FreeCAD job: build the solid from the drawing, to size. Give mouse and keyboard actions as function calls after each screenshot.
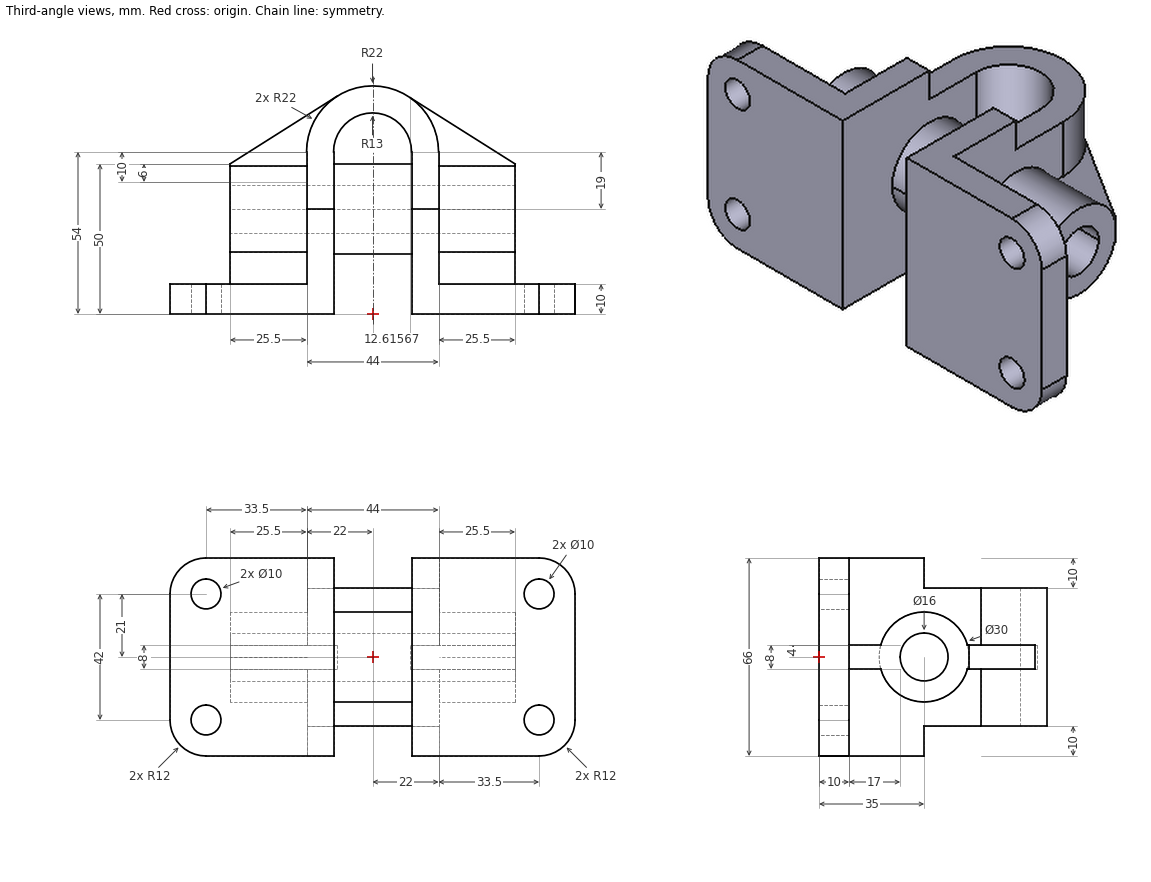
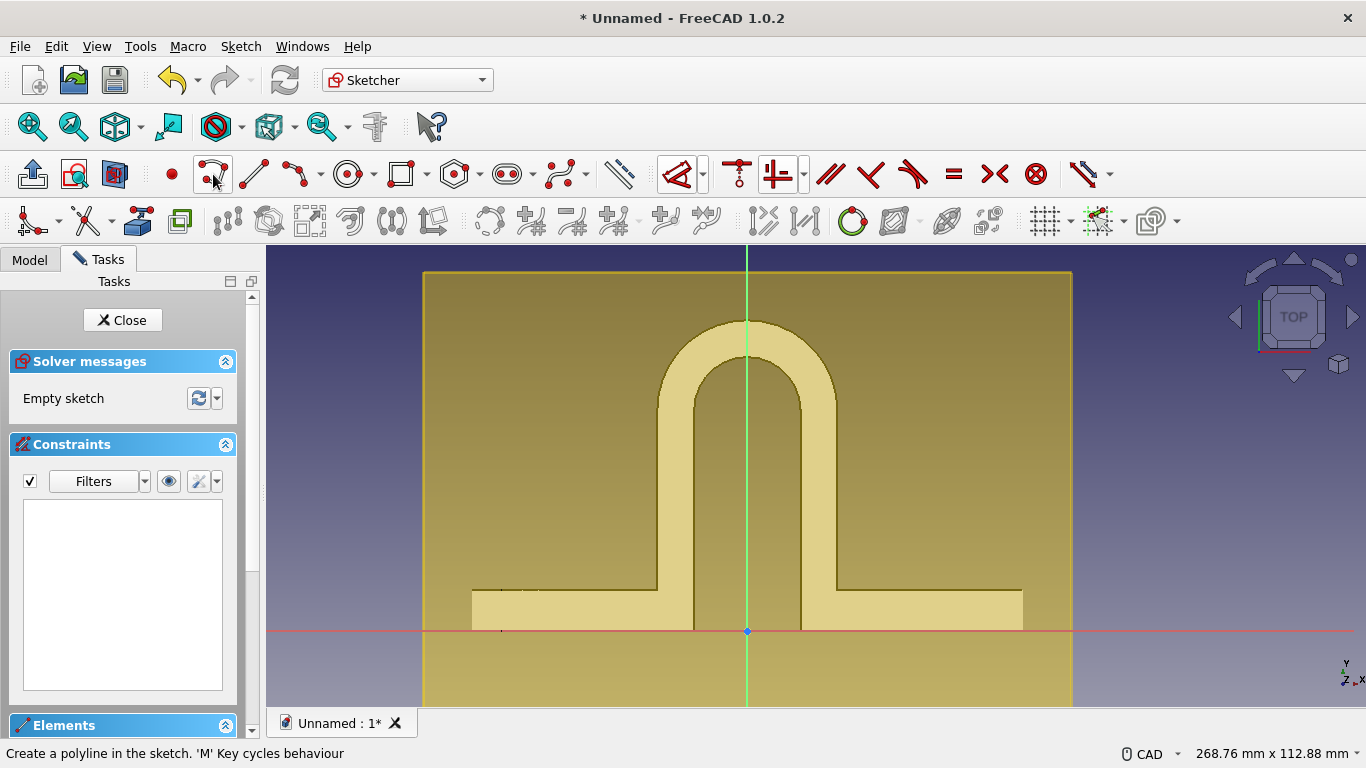
click(694, 410)
click(694, 488)
click(657, 488)
click(657, 410)
right_click(657, 410)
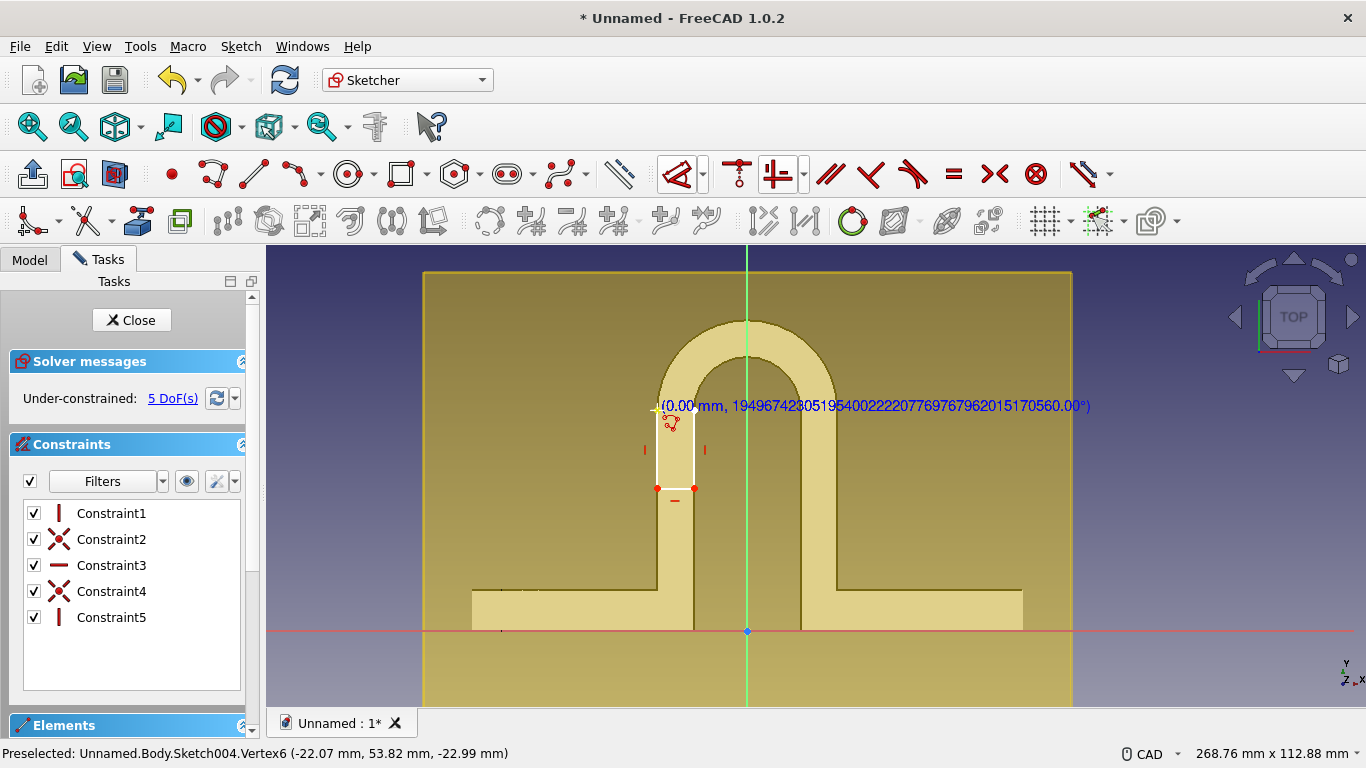
click(837, 410)
click(837, 488)
click(801, 488)
click(801, 410)
right_click(801, 410)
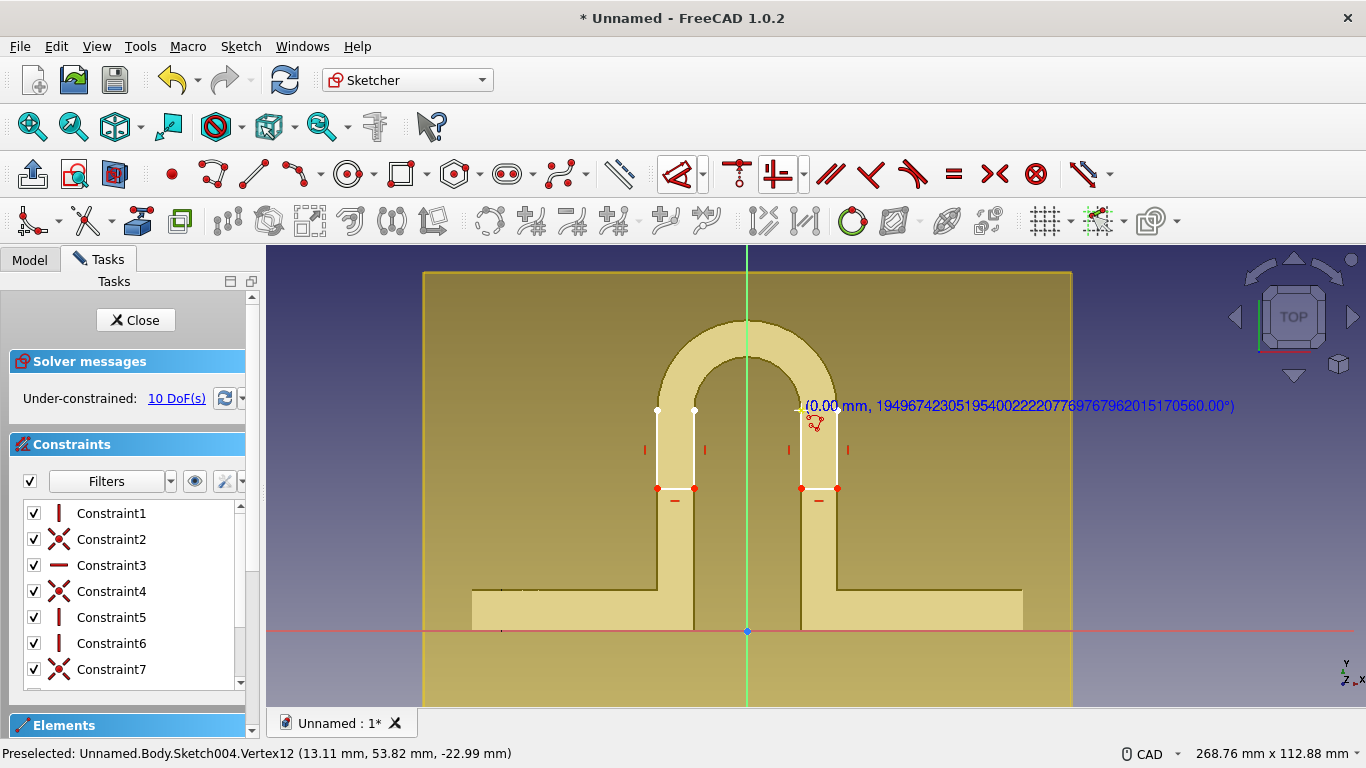
click(294, 174)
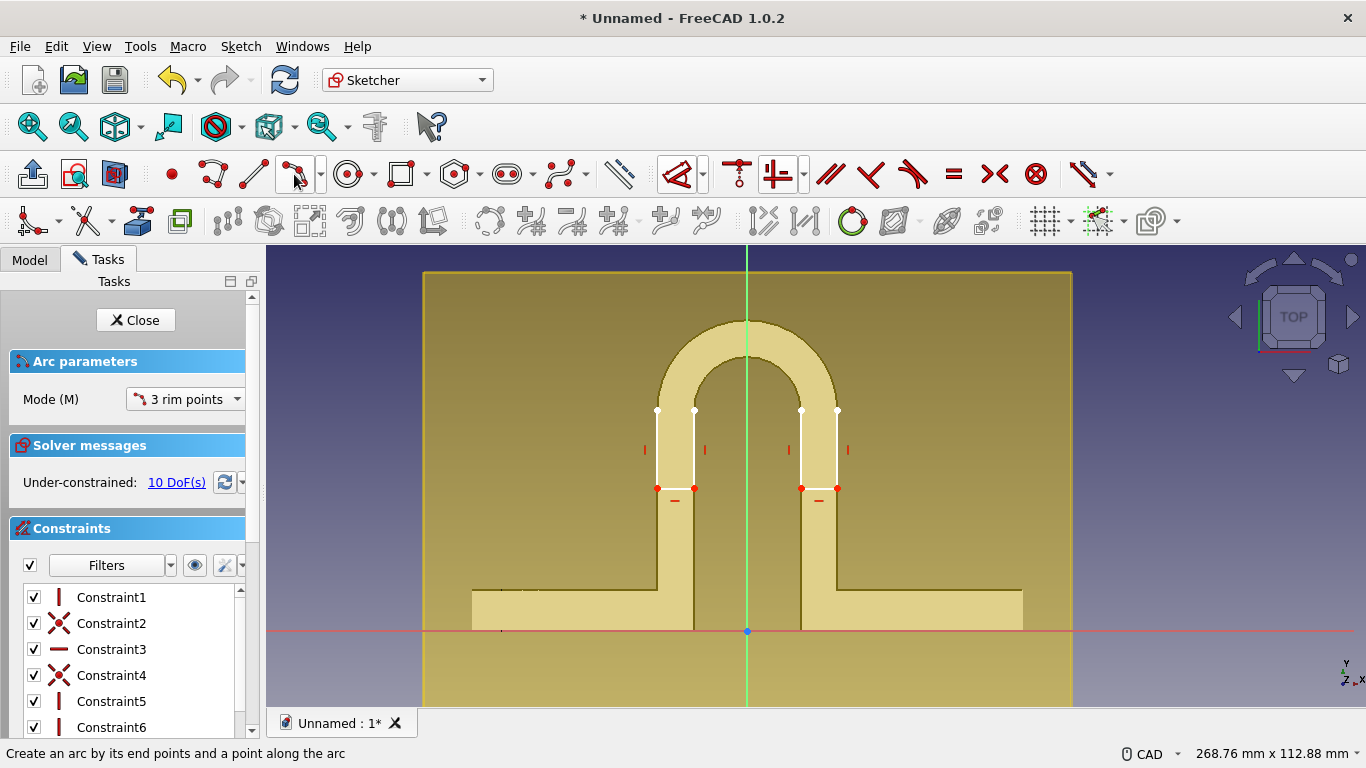
click(657, 411)
click(837, 411)
click(775, 325)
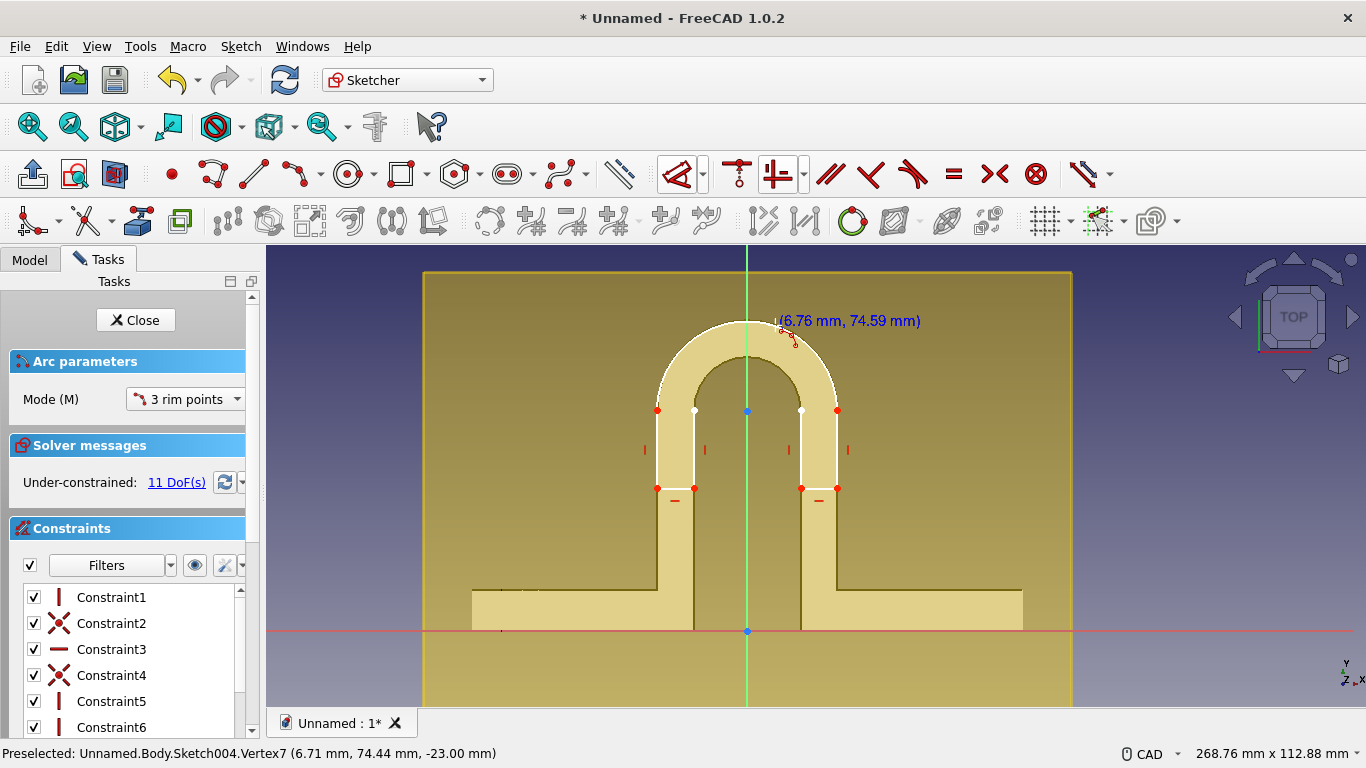
click(801, 411)
click(694, 411)
click(764, 360)
key(Escape)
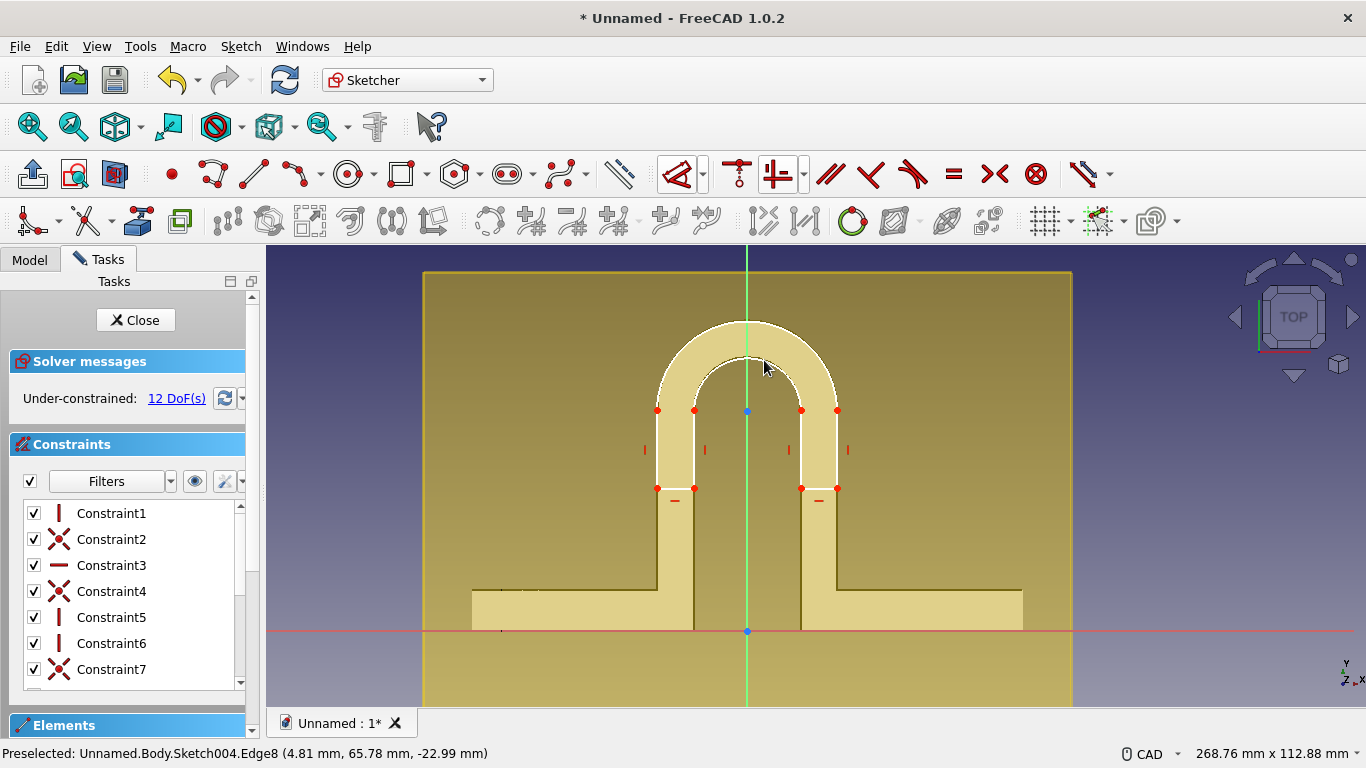
click(694, 434)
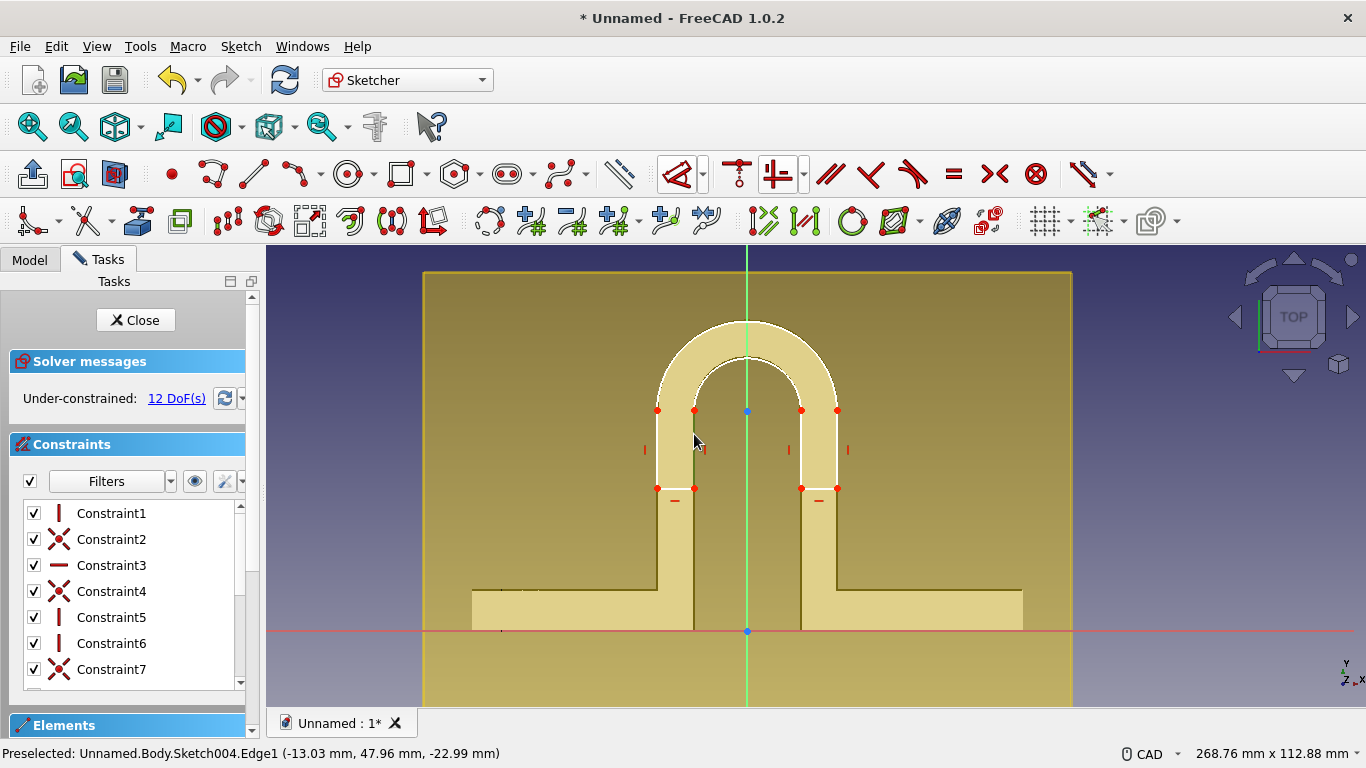
click(779, 368)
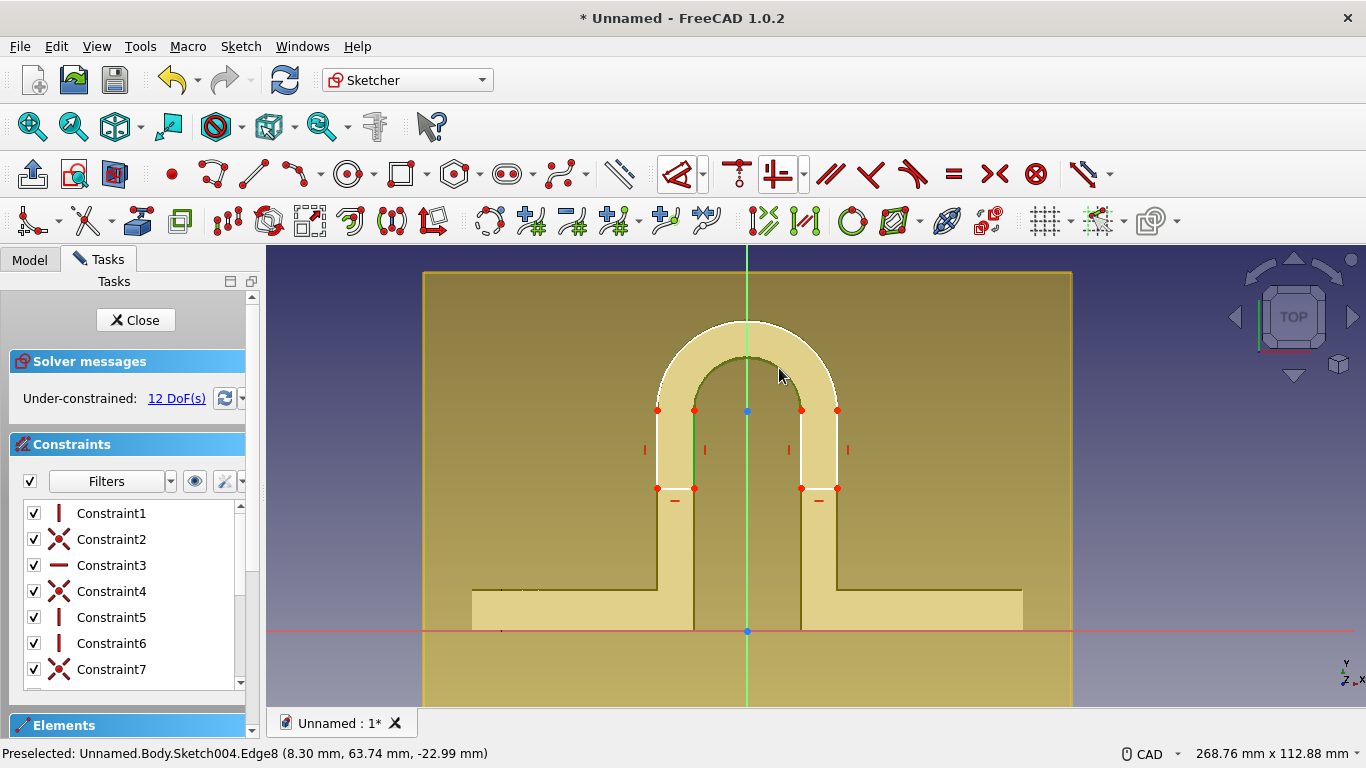
click(913, 174)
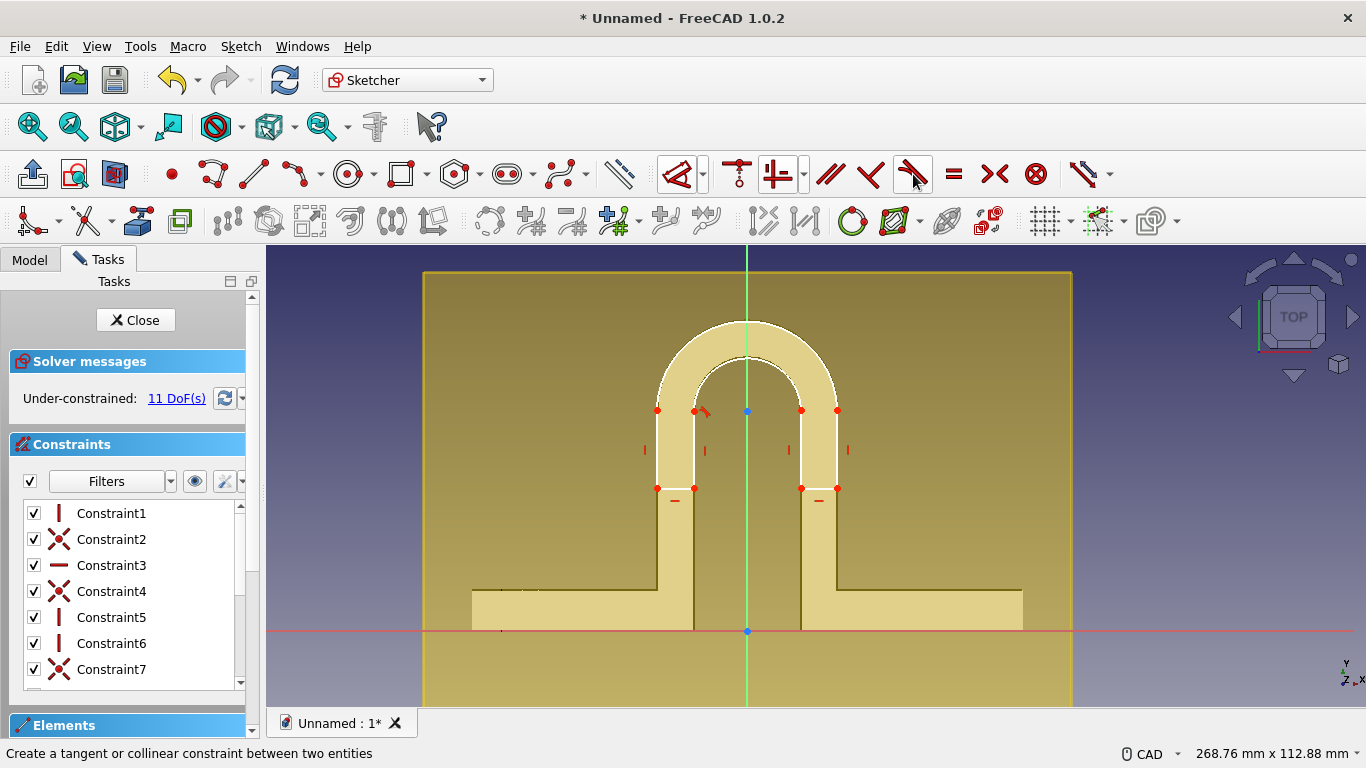
click(657, 466)